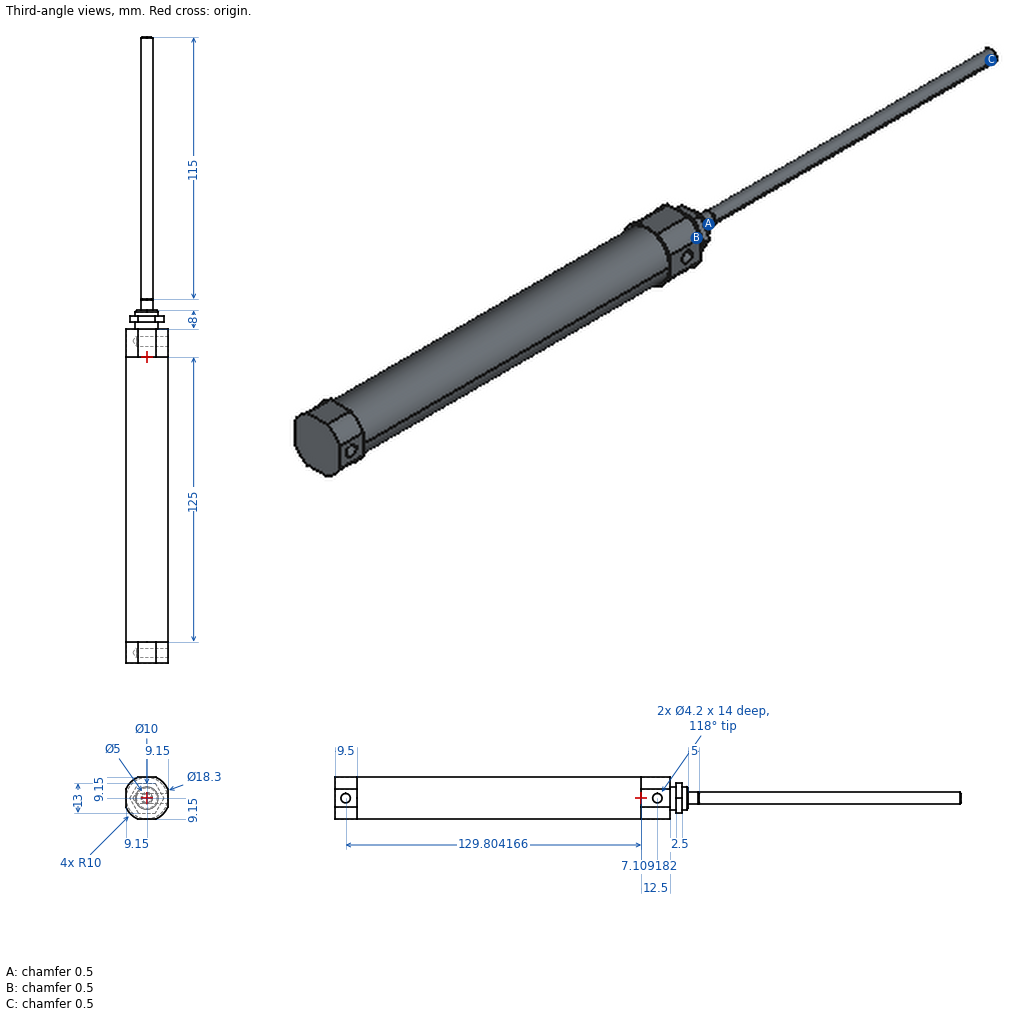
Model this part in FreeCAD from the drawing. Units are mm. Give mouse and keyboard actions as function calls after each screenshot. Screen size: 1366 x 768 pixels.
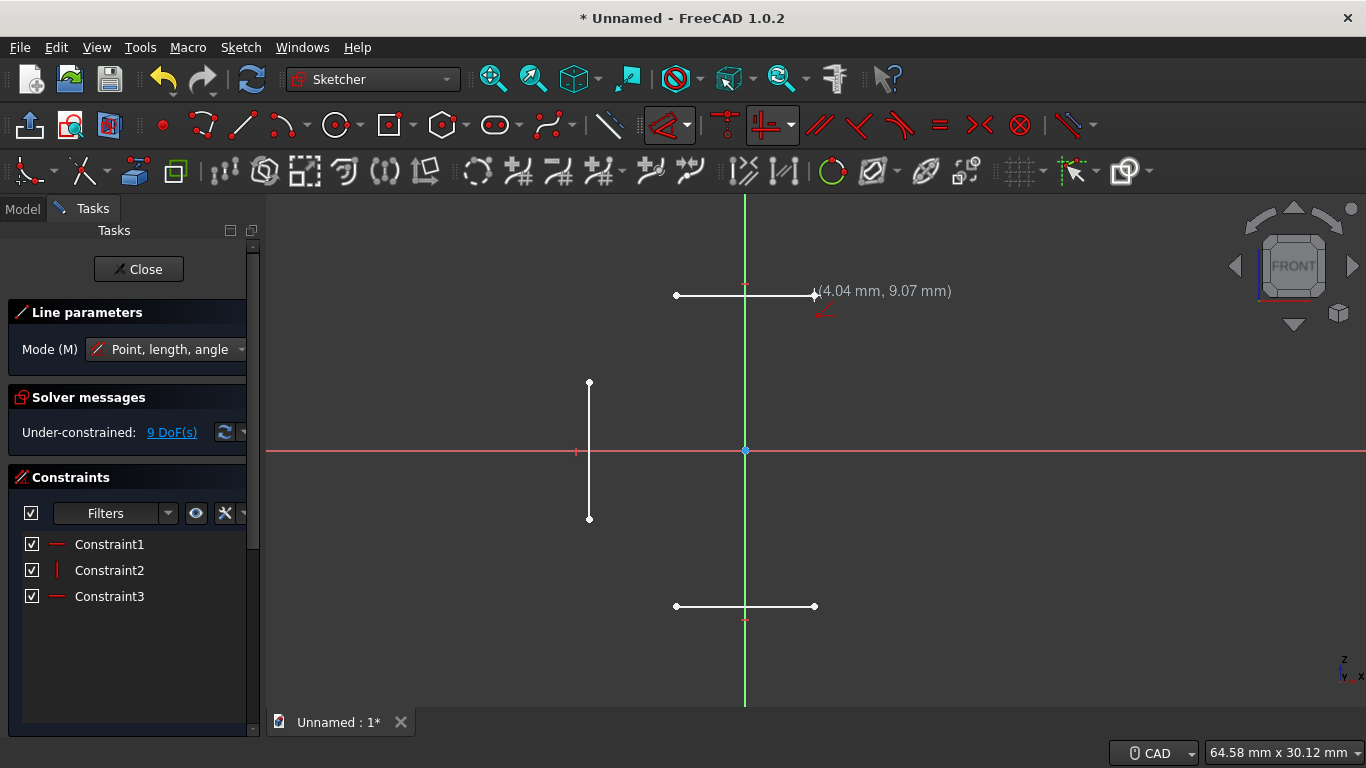
click(901, 382)
click(901, 519)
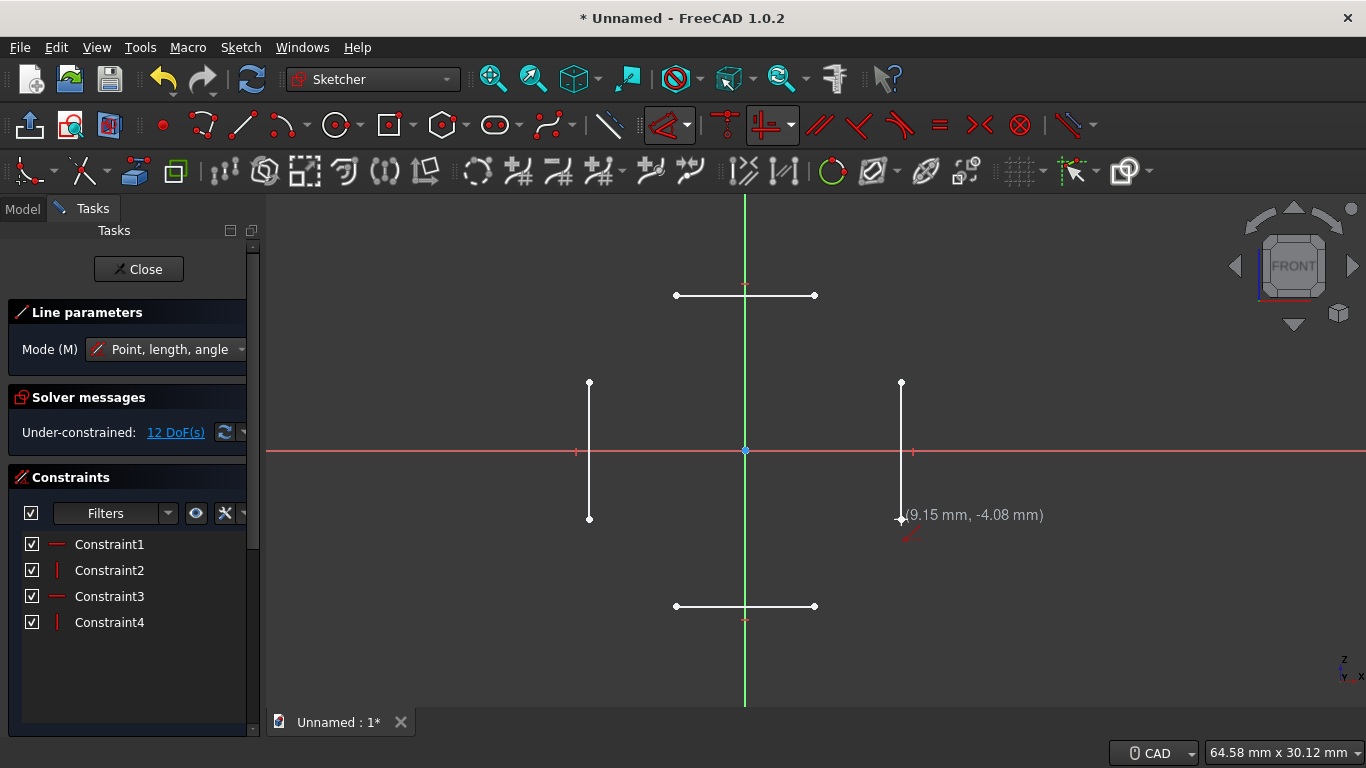
key(g)
key(3)
key(a)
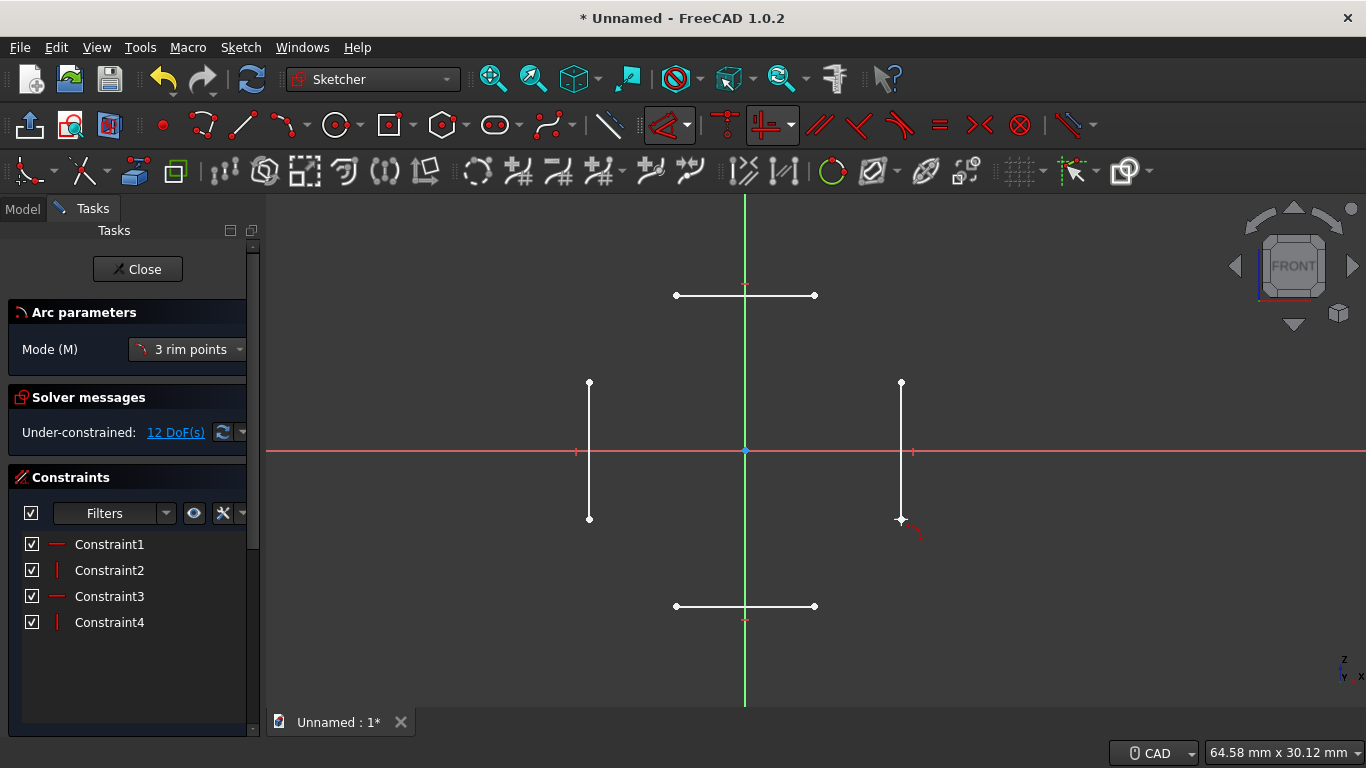
click(676, 607)
click(589, 520)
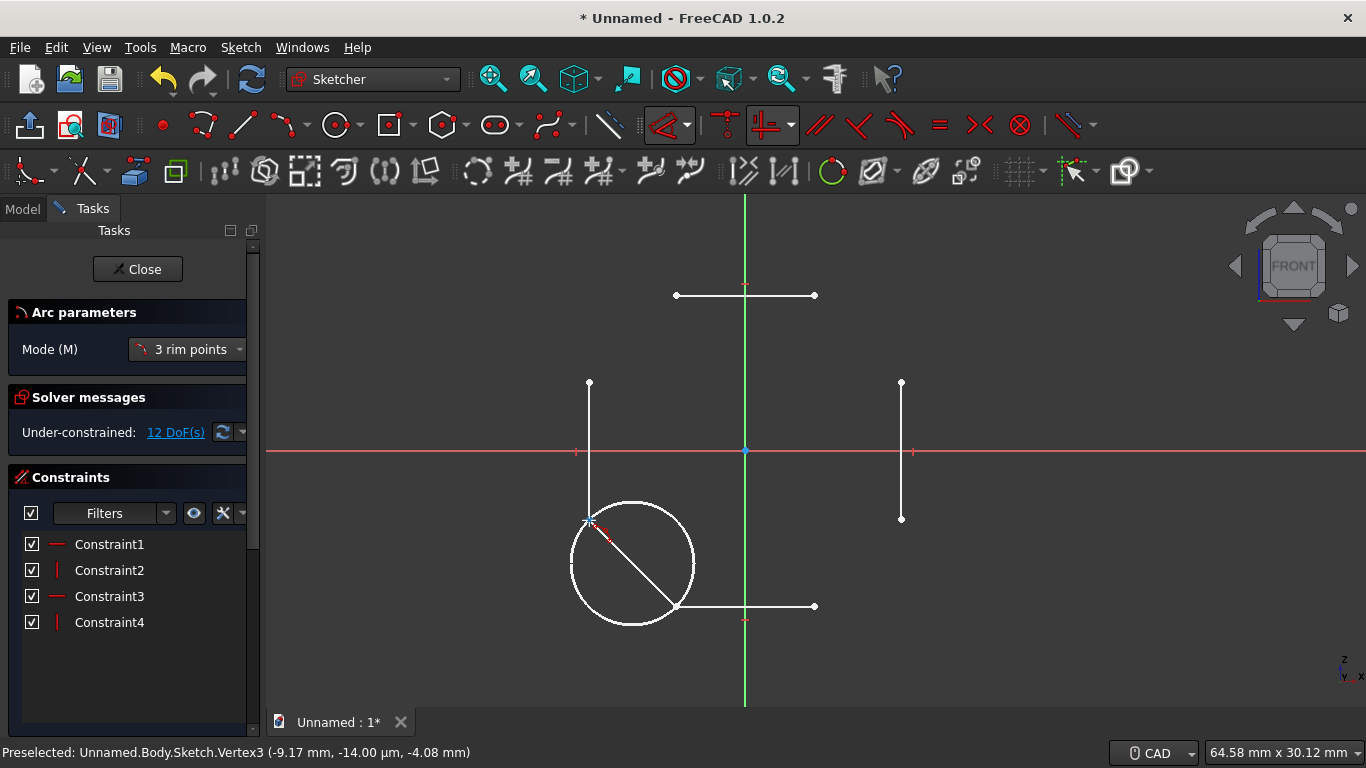
scroll(625, 571, up, 2)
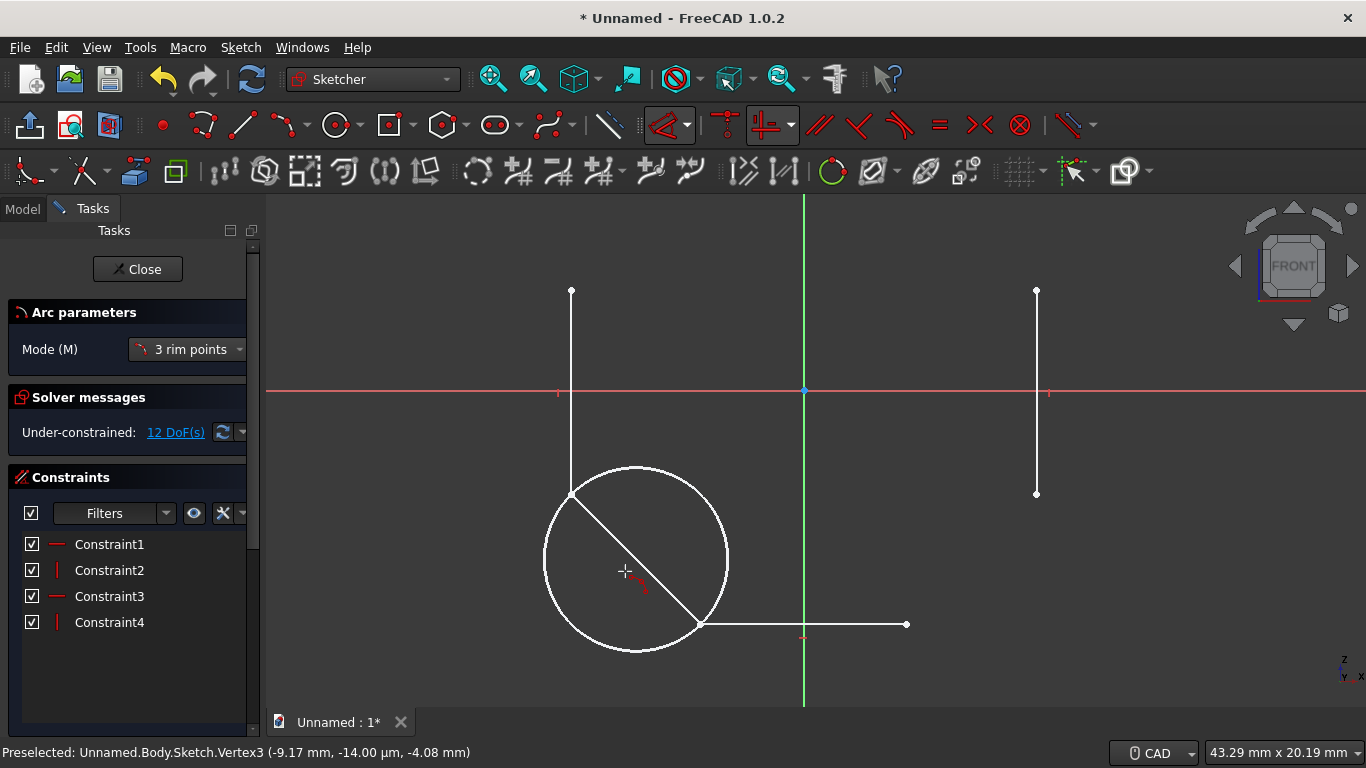
click(624, 571)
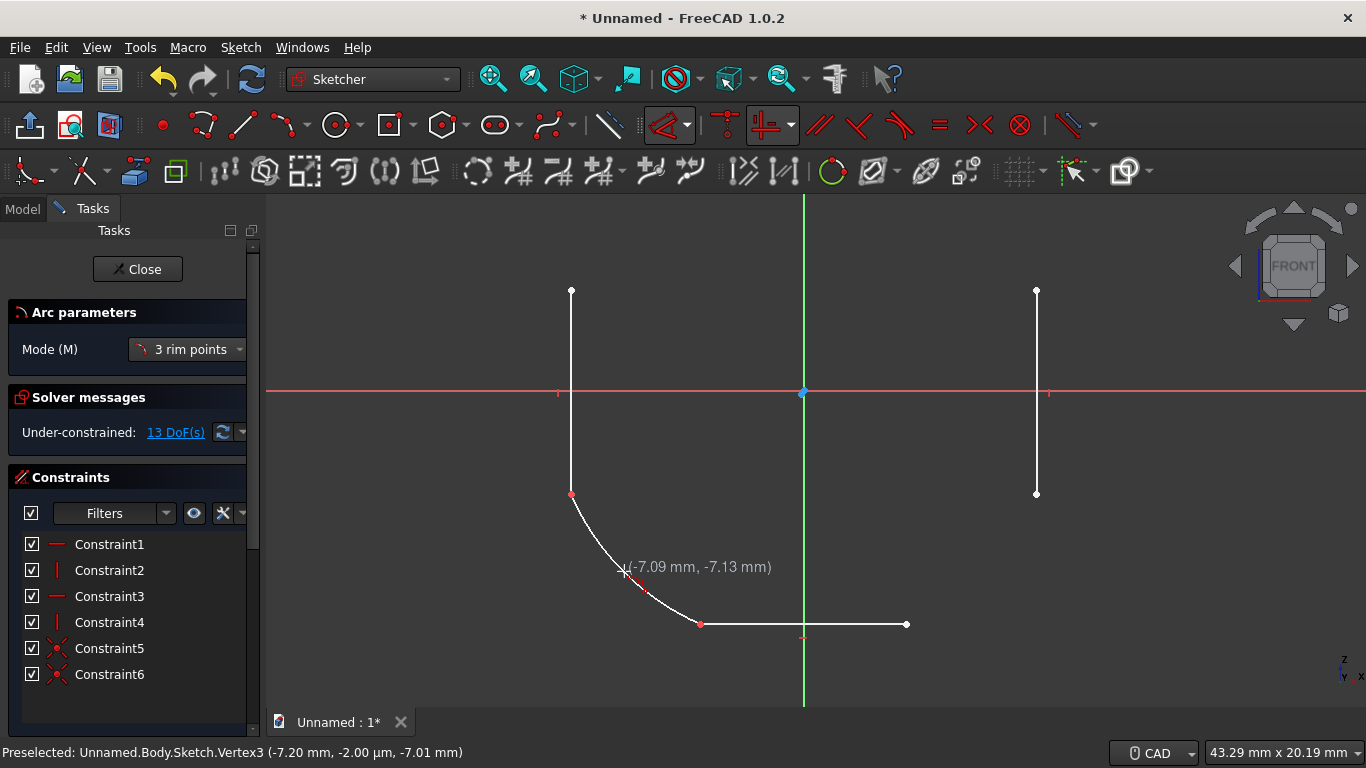
click(571, 290)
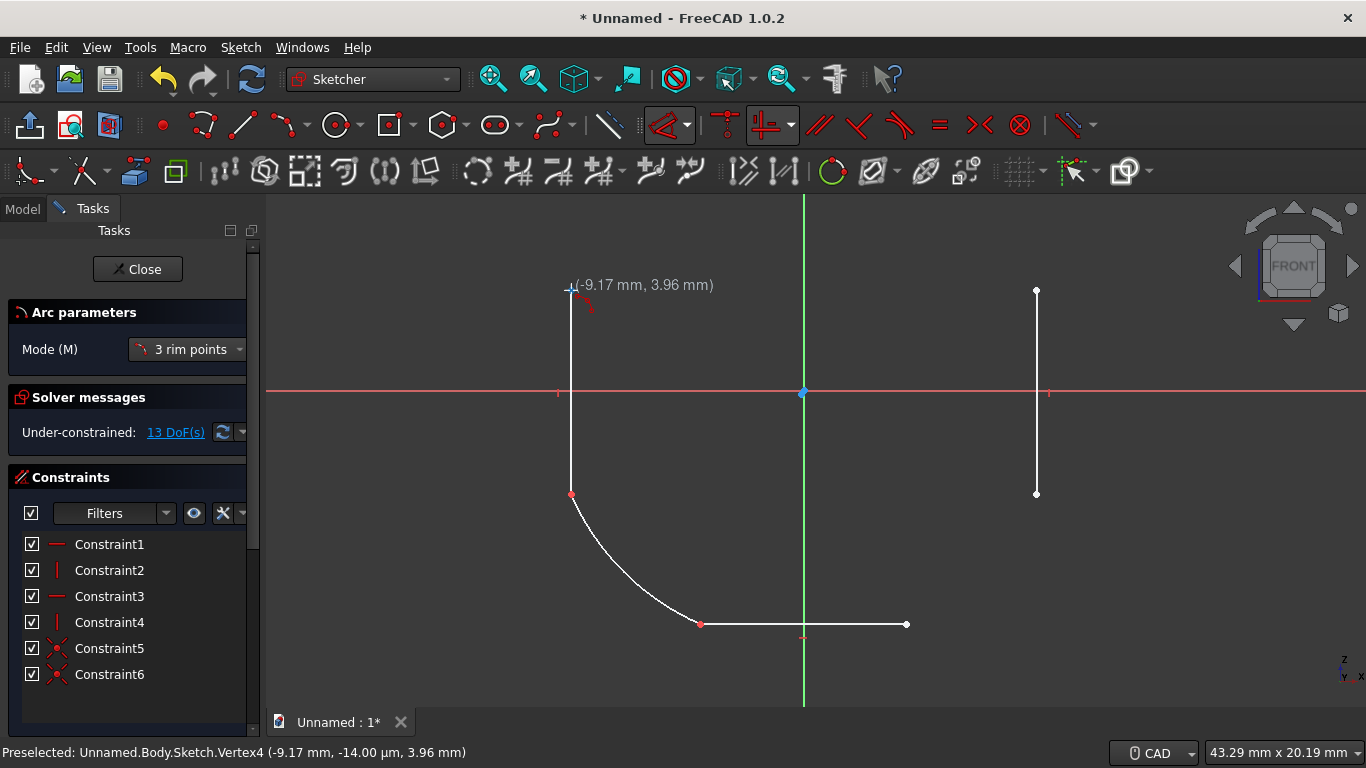
scroll(632, 572, down, 2)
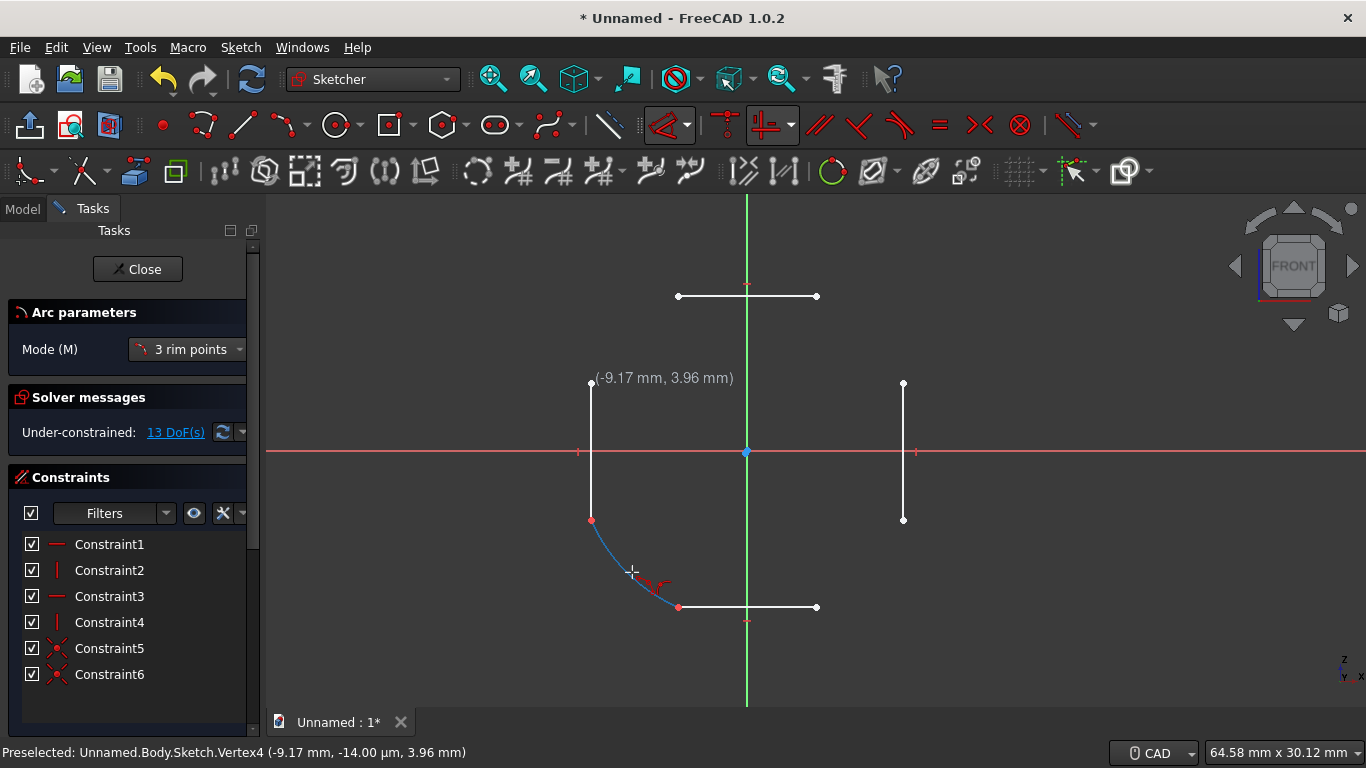
click(678, 296)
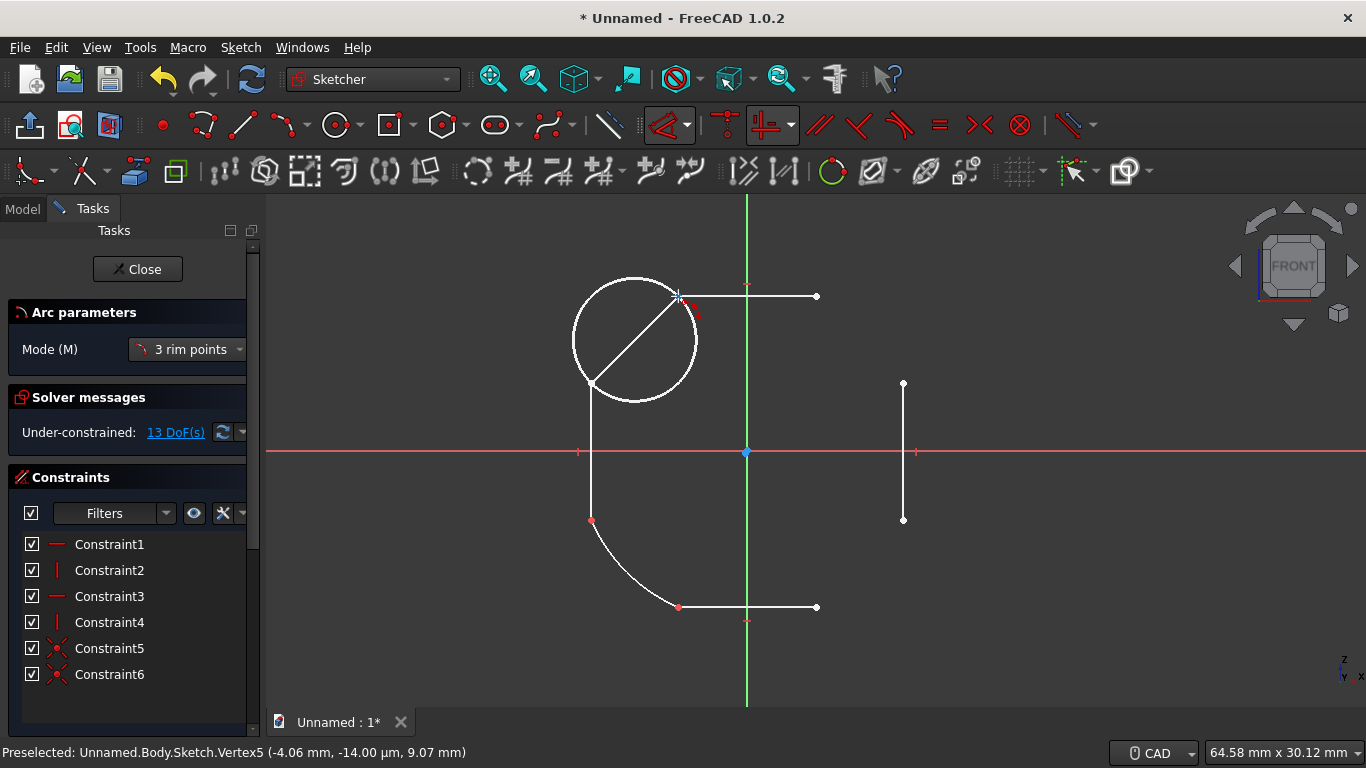
scroll(627, 330, up, 2)